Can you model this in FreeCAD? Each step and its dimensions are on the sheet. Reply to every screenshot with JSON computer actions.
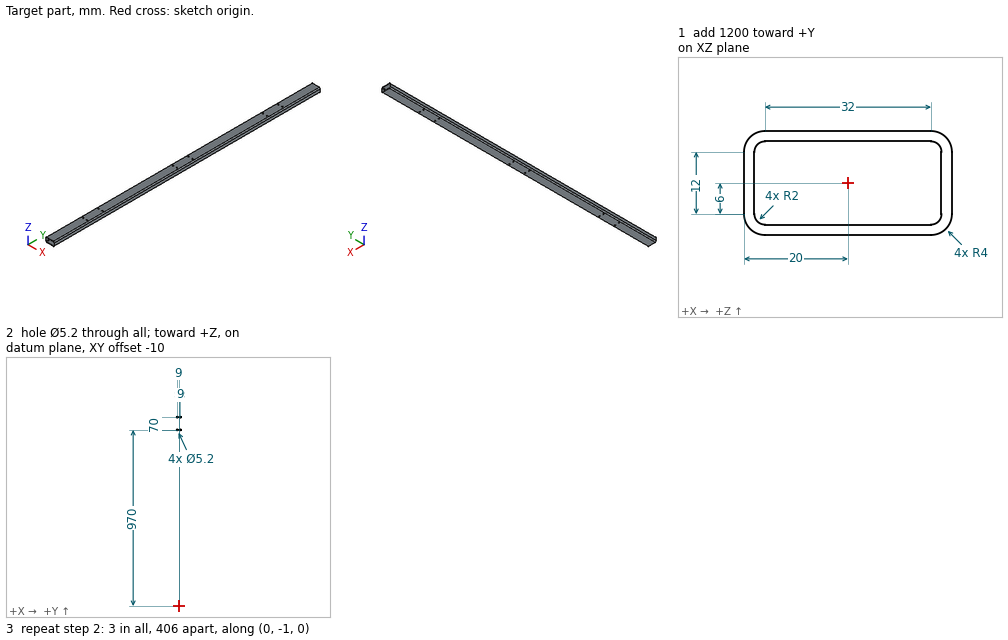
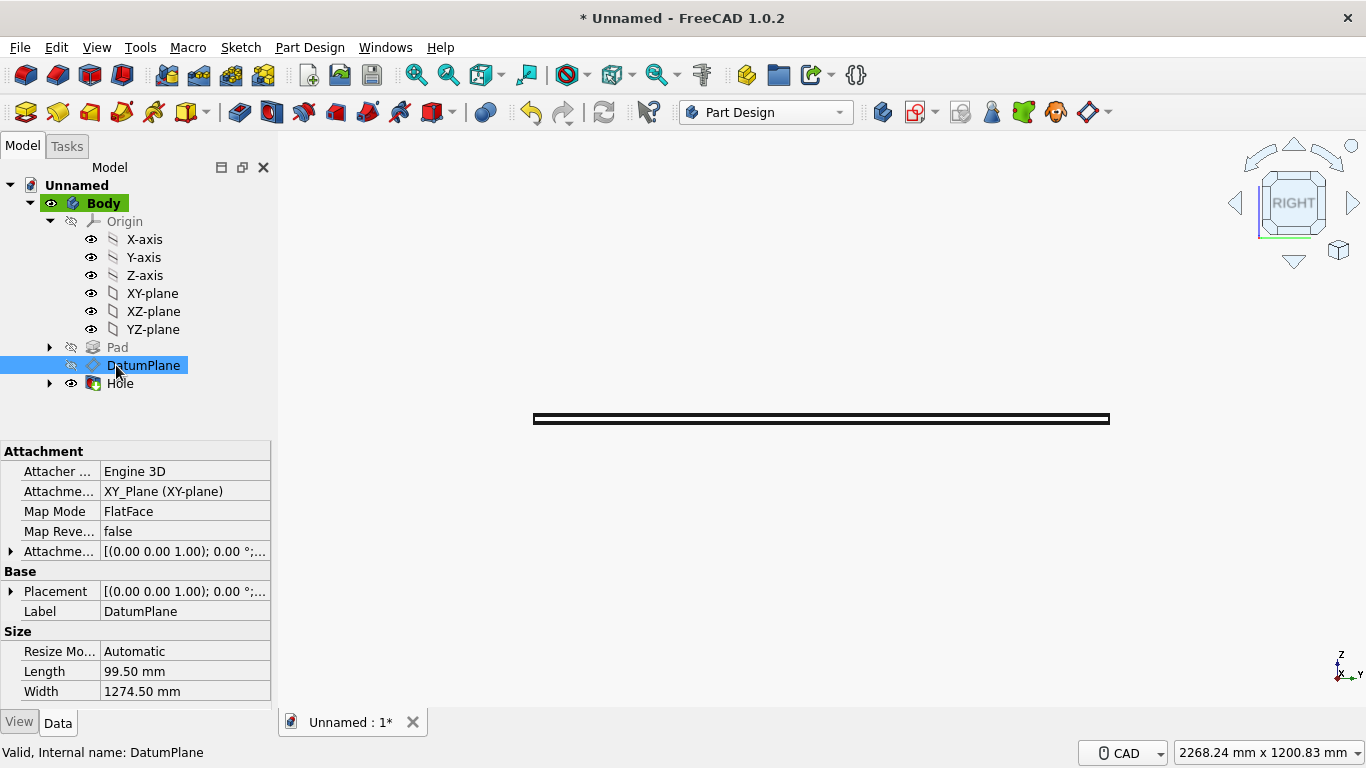
{"action": "left_click", "coordinate": [116, 383]}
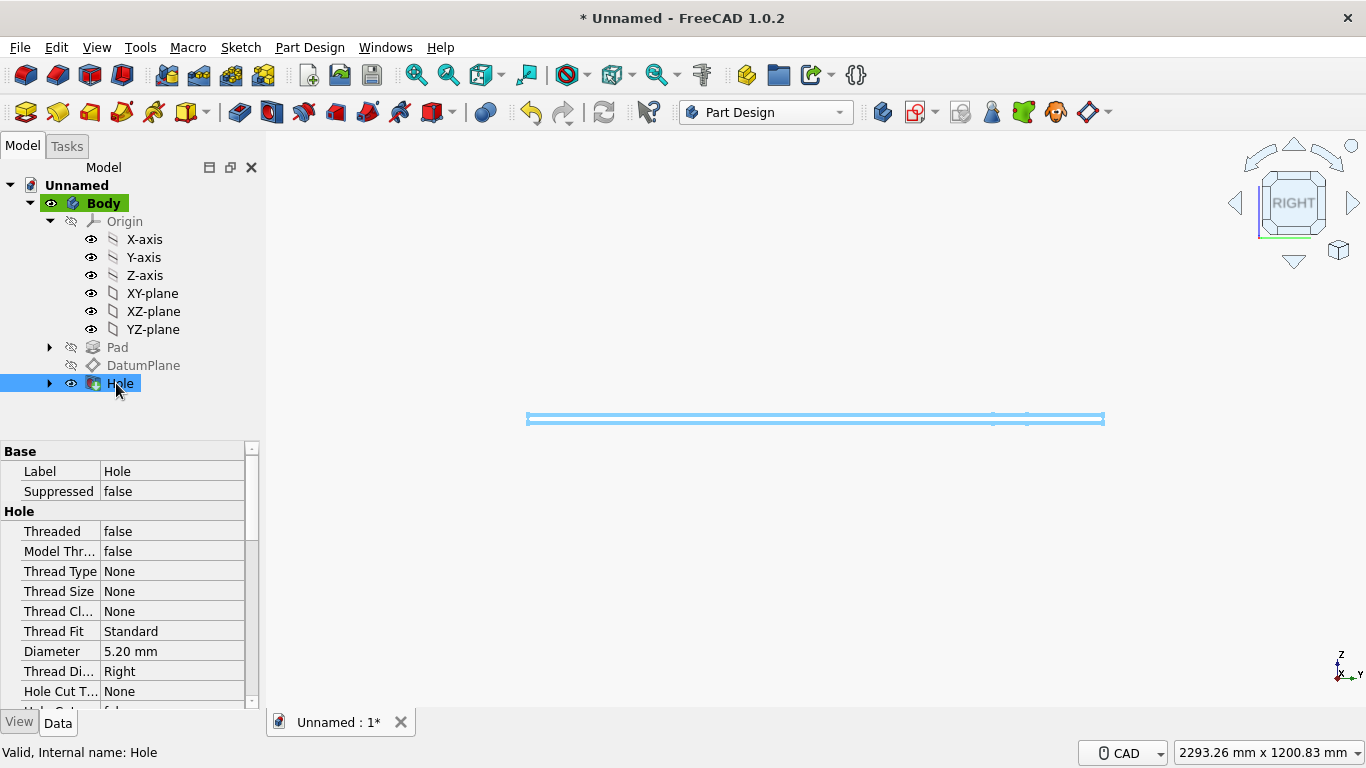
{"action": "left_click", "coordinate": [200, 76]}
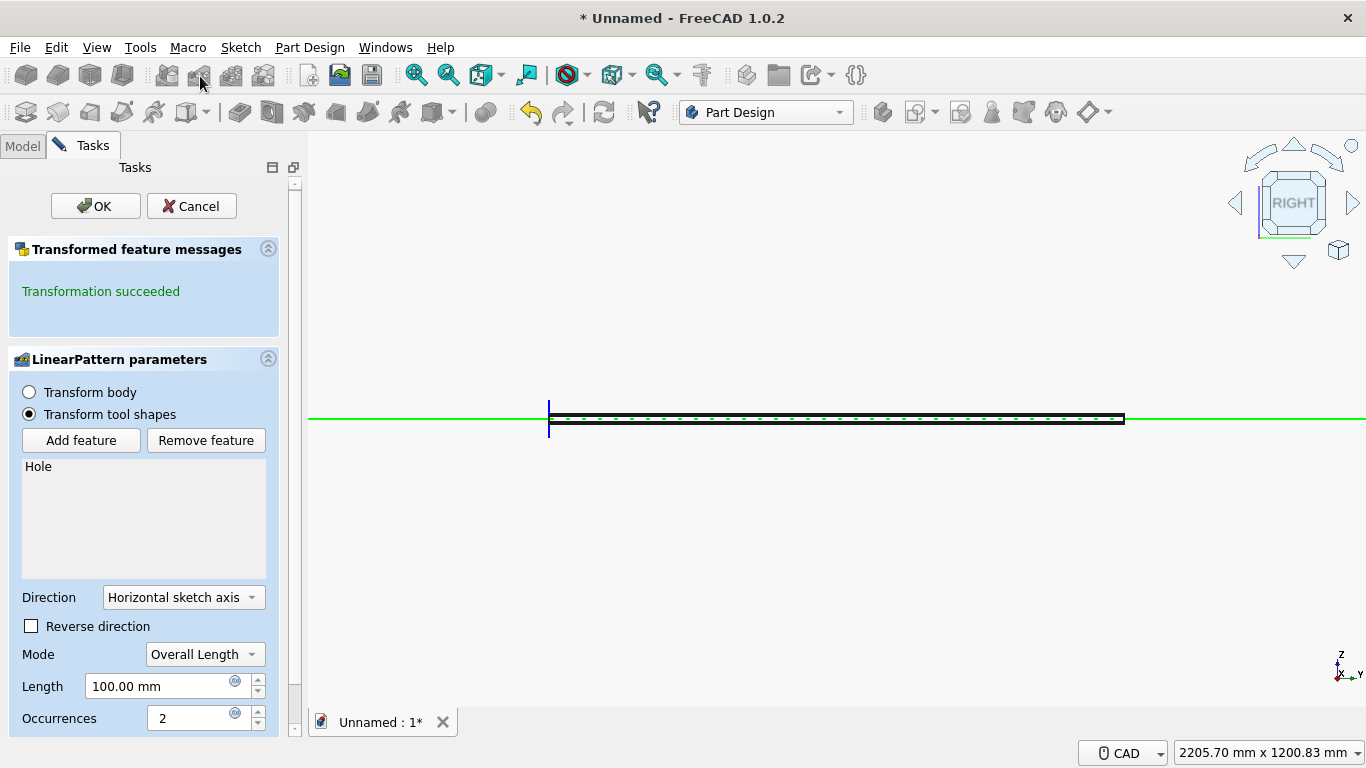
{"action": "left_click", "coordinate": [184, 598]}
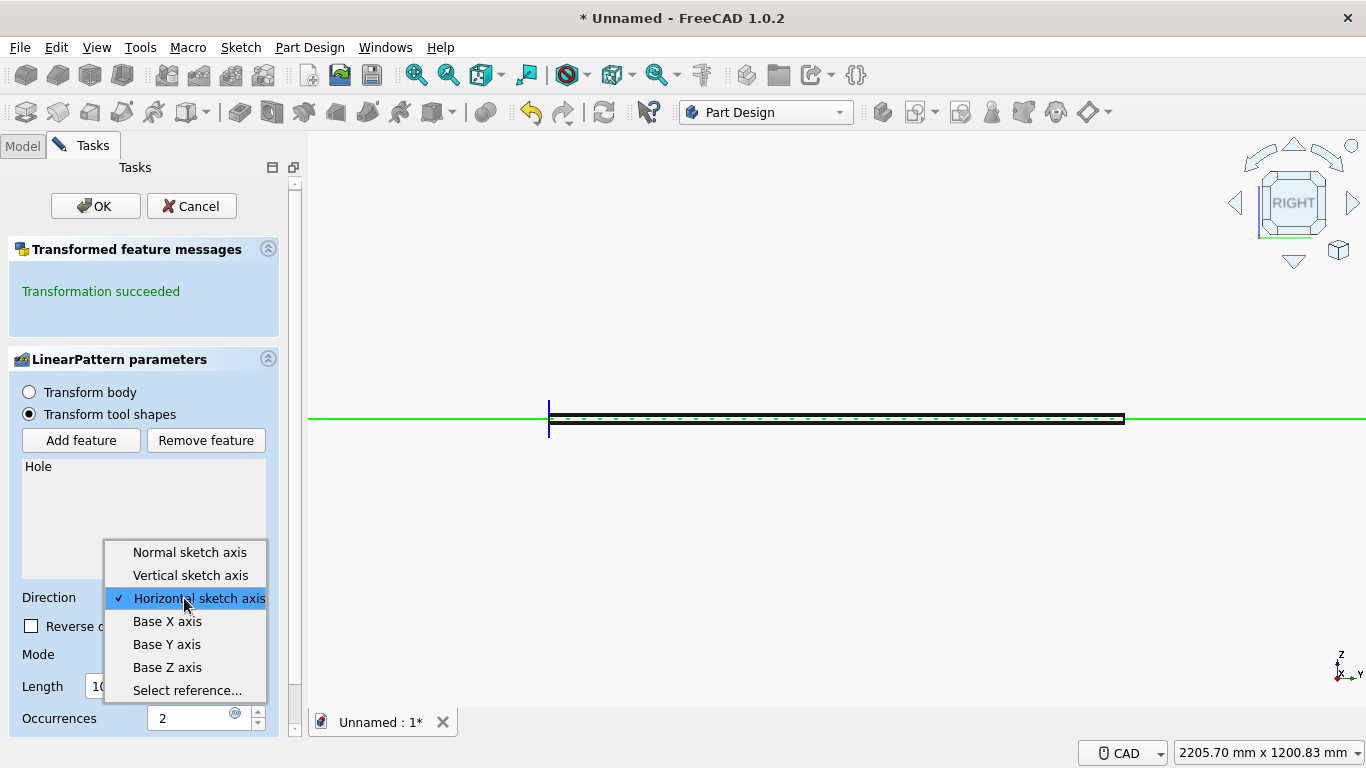
{"action": "left_click", "coordinate": [184, 644]}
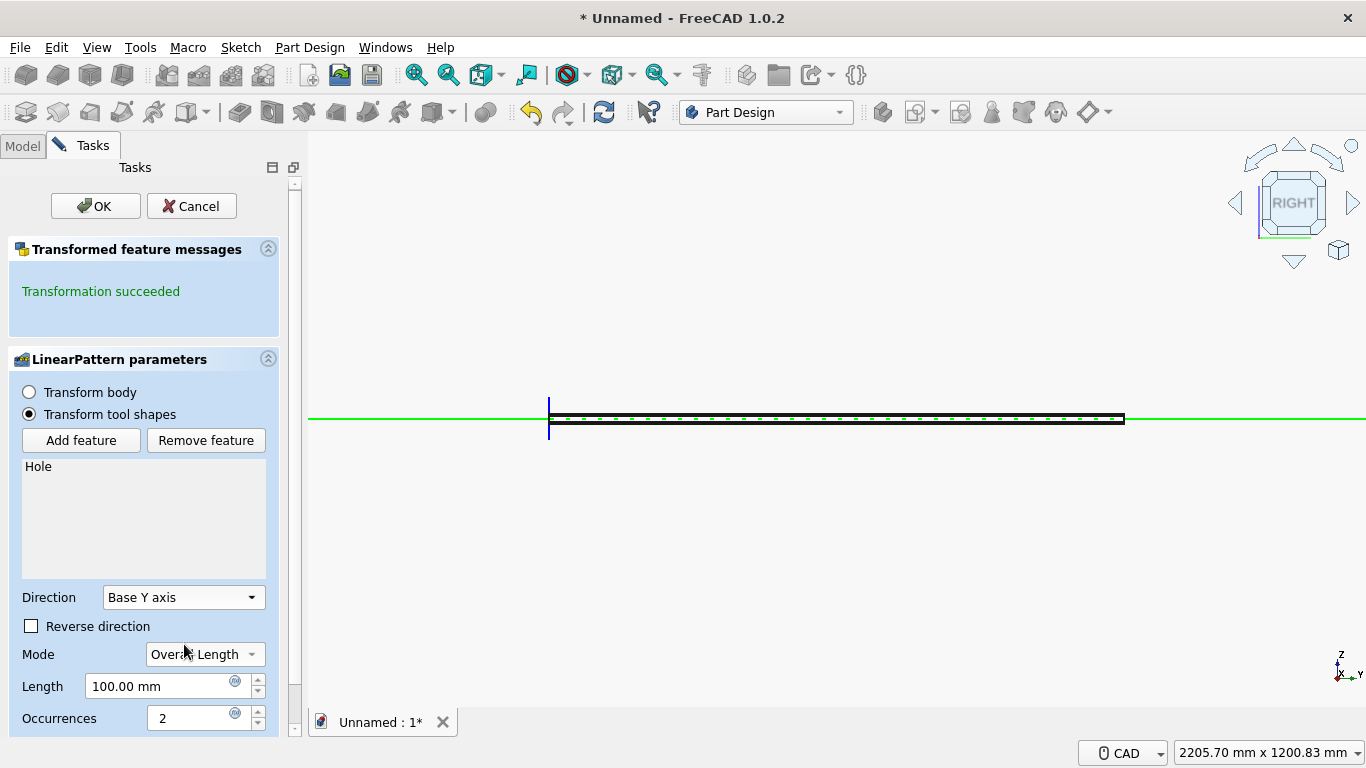
{"action": "left_click", "coordinate": [206, 654]}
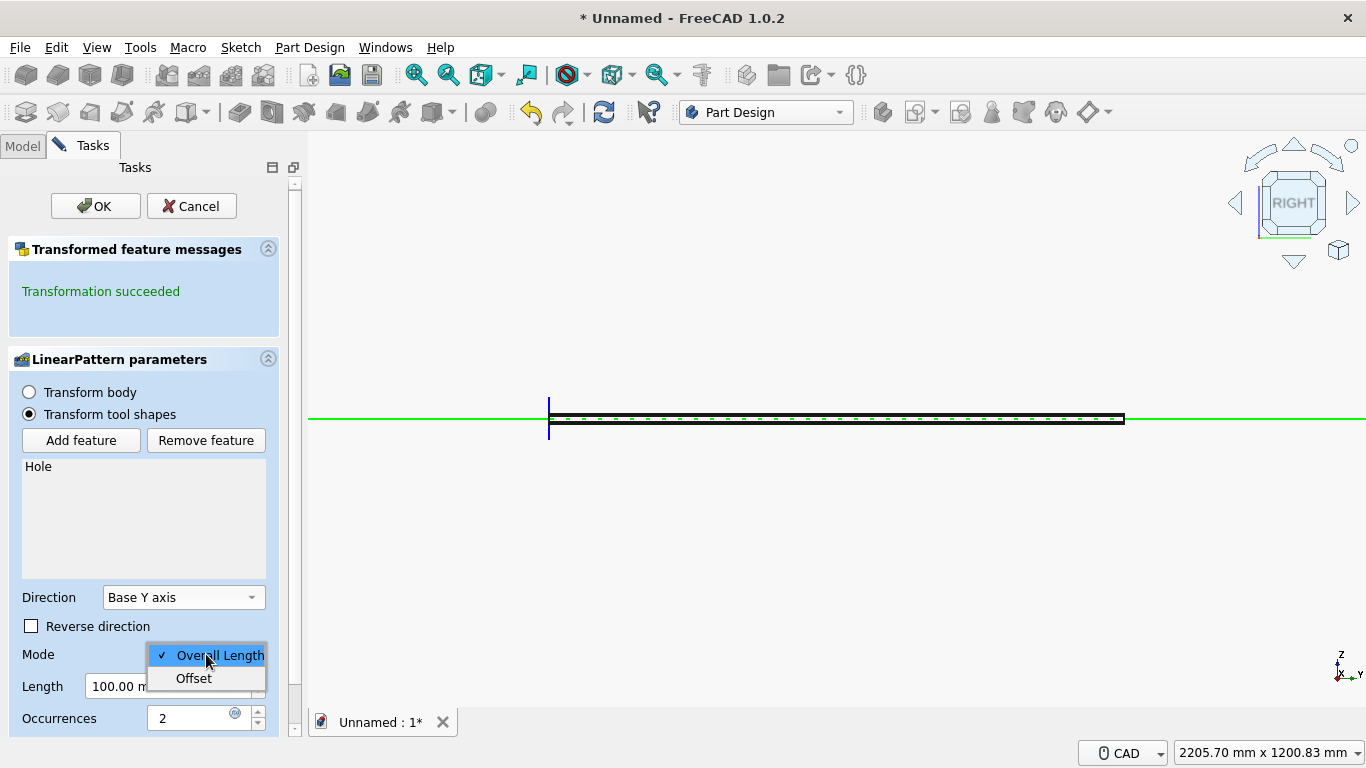
{"action": "left_click", "coordinate": [206, 678]}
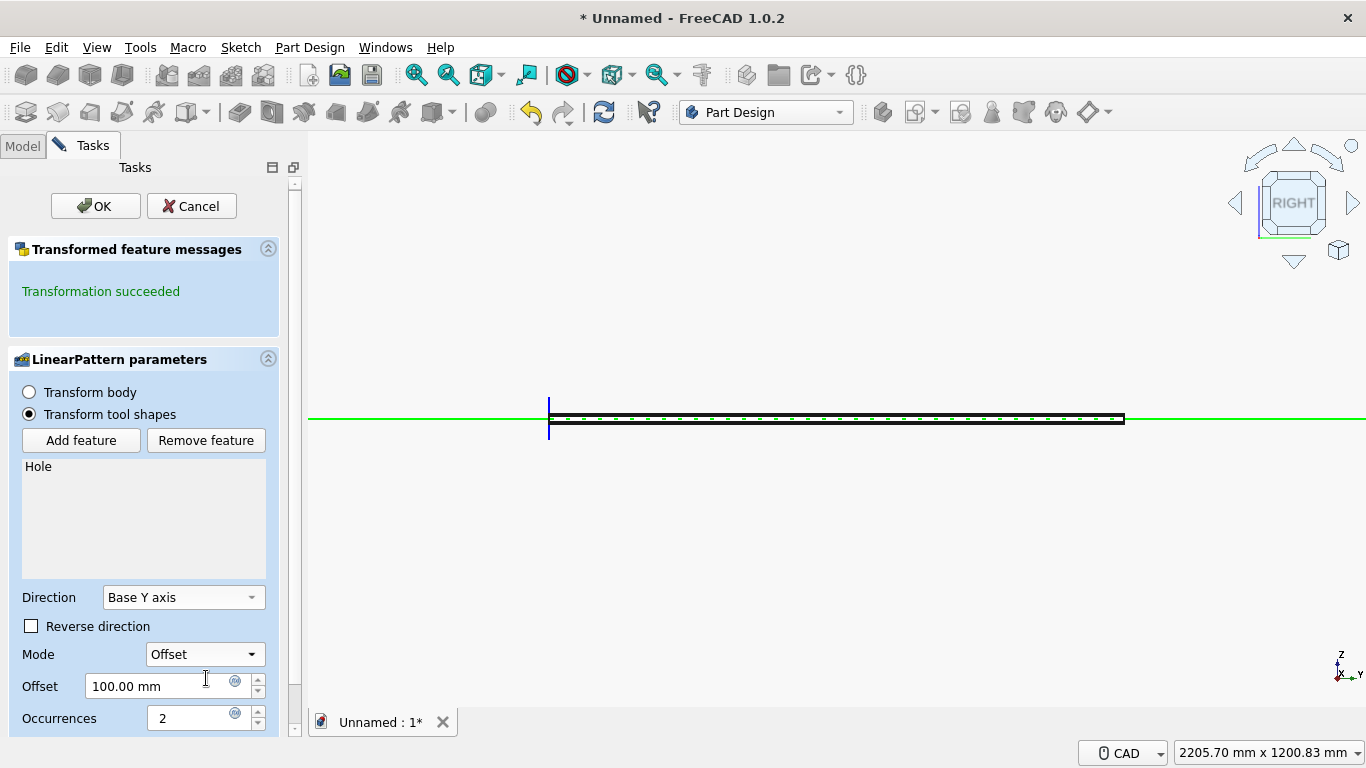
{"action": "triple_click", "coordinate": [168, 686]}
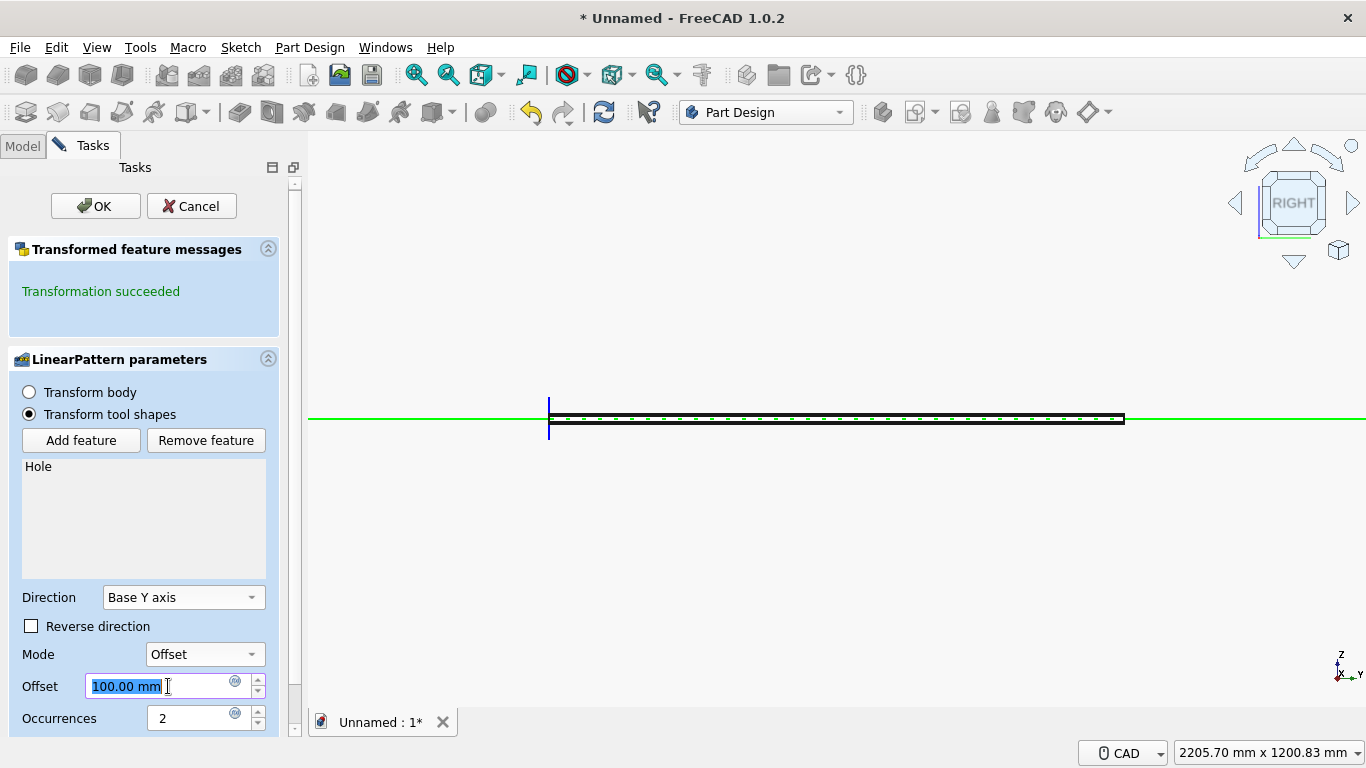
{"action": "type", "text": "406"}
{"action": "key", "text": "Tab"}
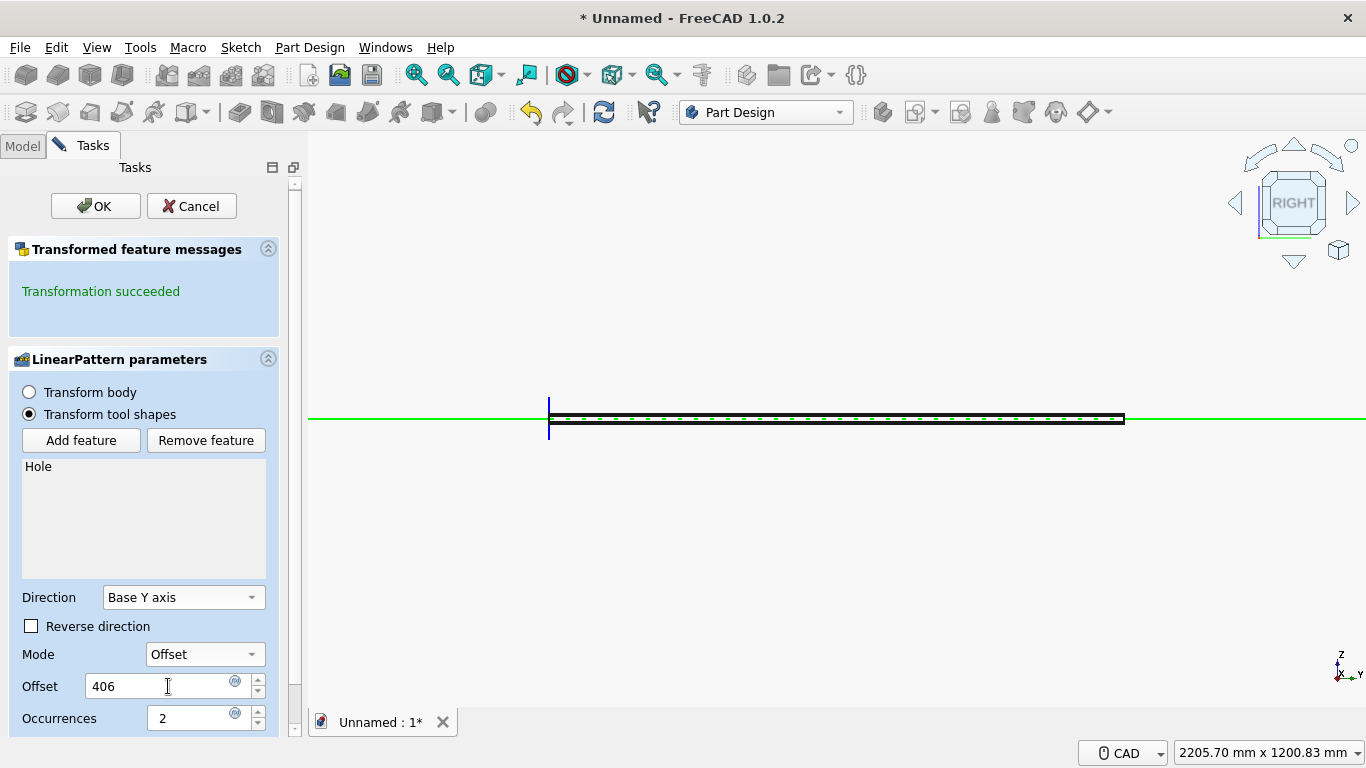
{"action": "triple_click", "coordinate": [198, 718]}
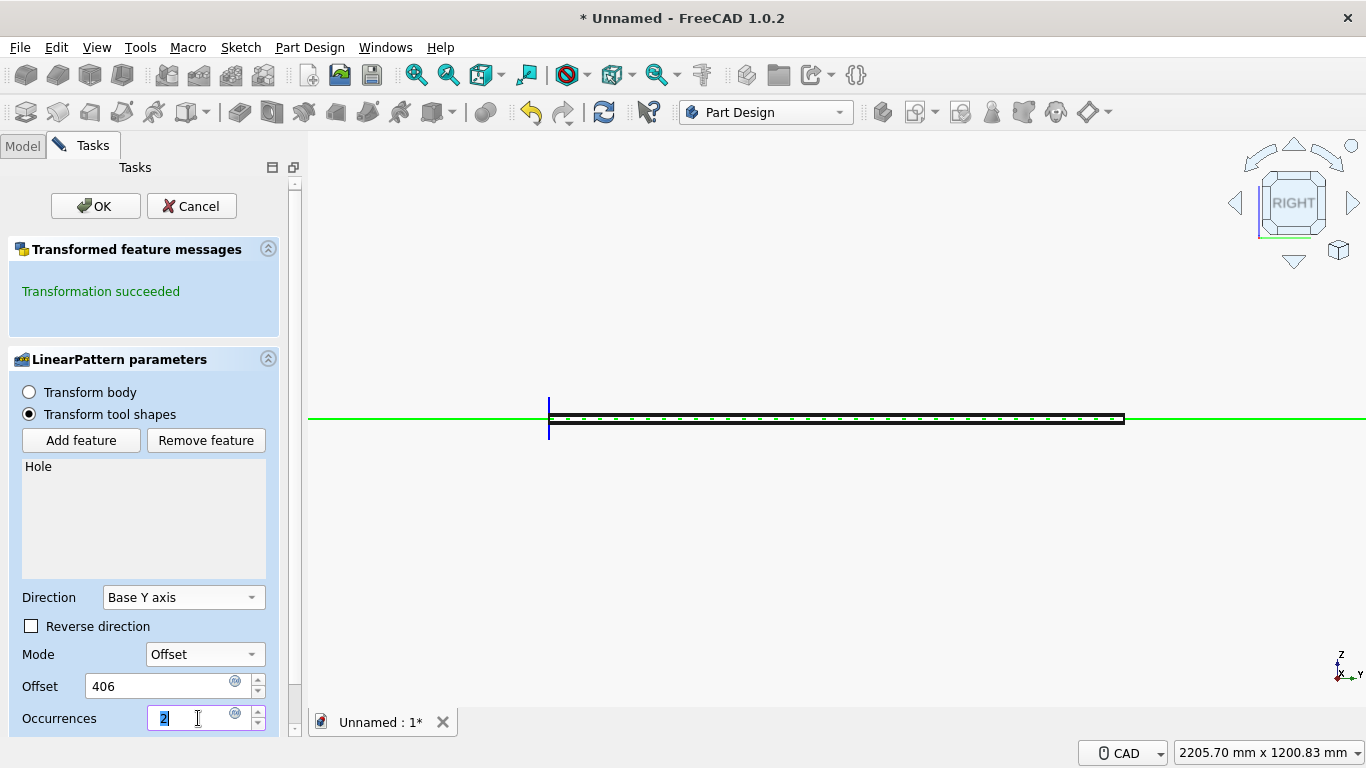
{"action": "type", "text": "3"}
{"action": "key", "text": "Tab"}